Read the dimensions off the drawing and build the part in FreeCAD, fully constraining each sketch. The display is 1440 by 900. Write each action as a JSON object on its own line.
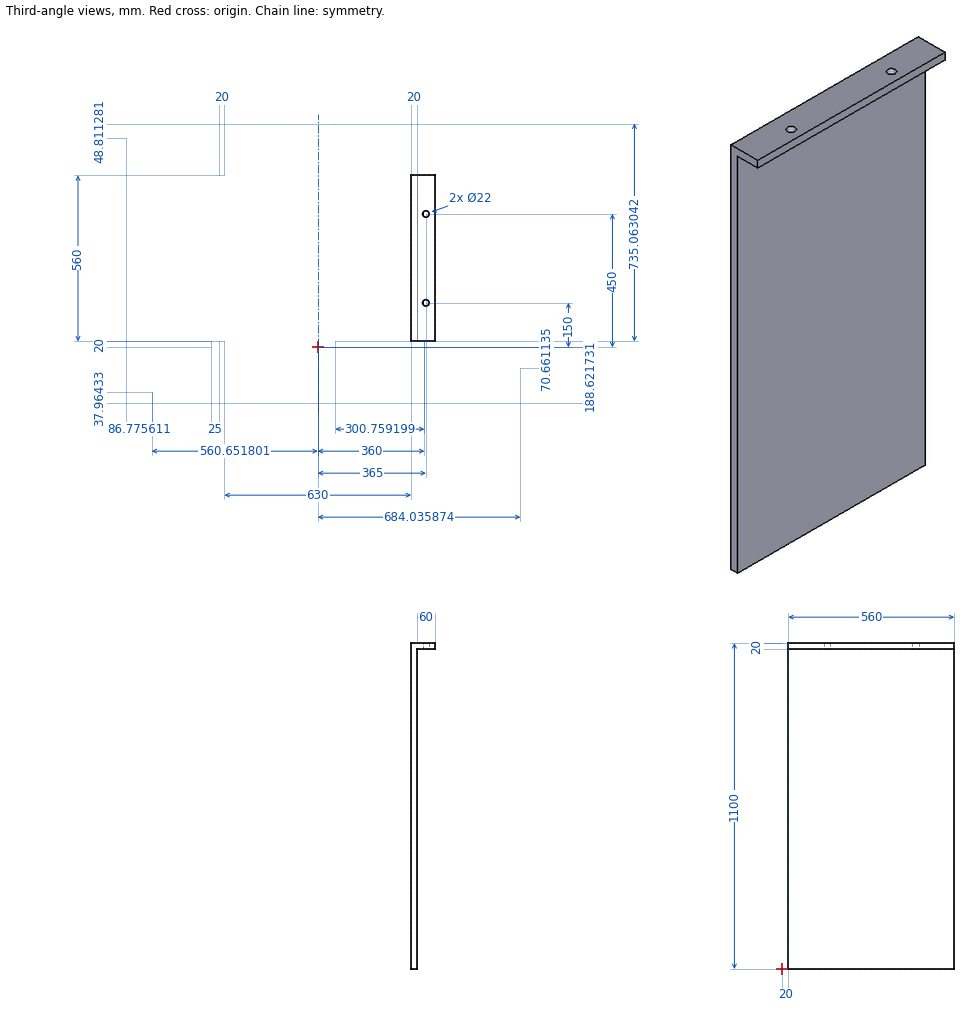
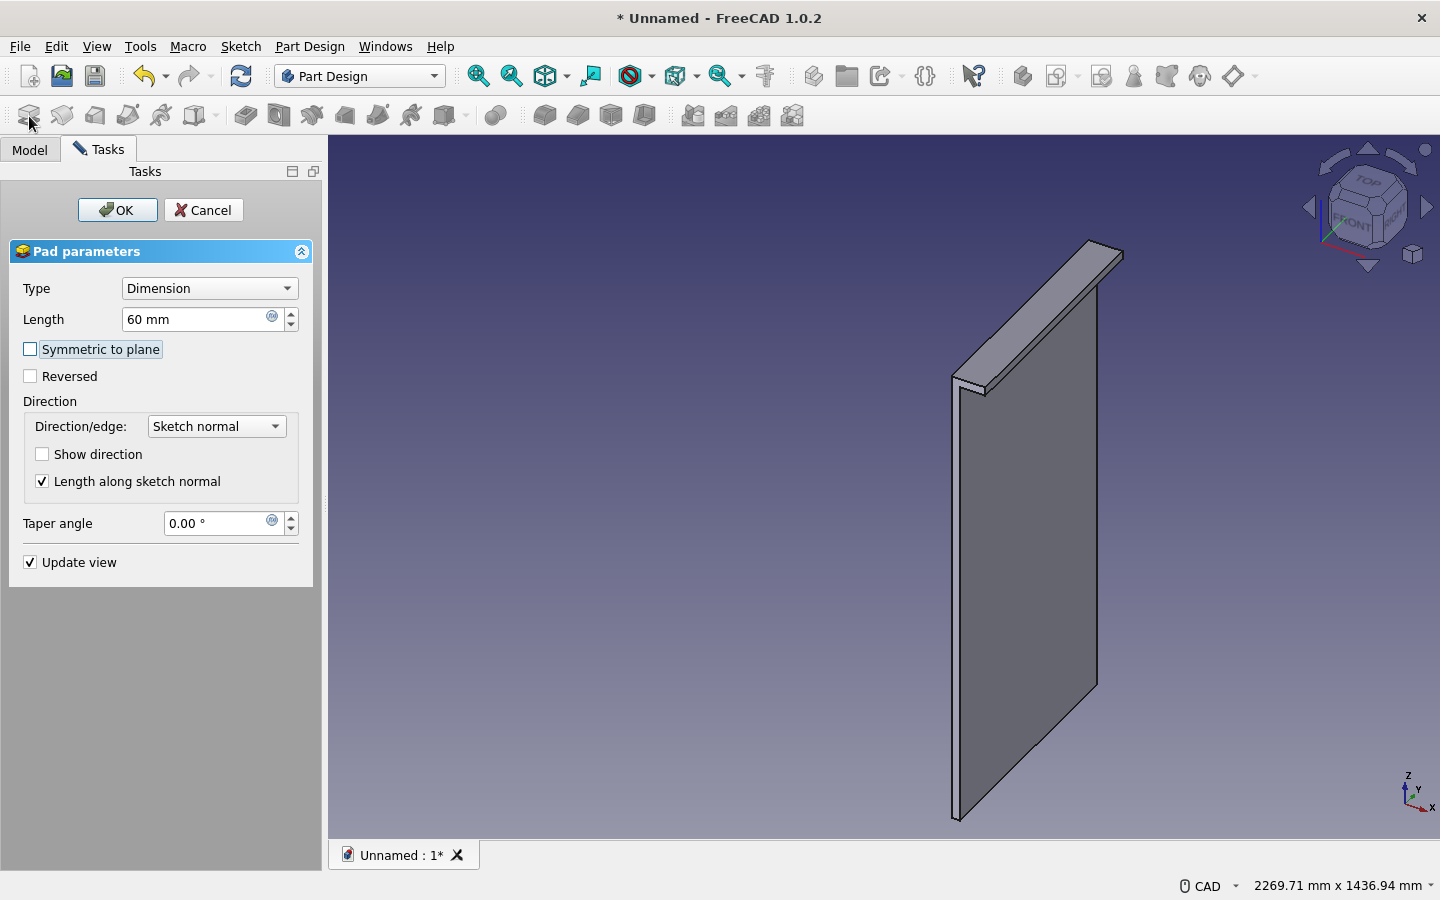
{"action": "left_click", "coordinate": [118, 210]}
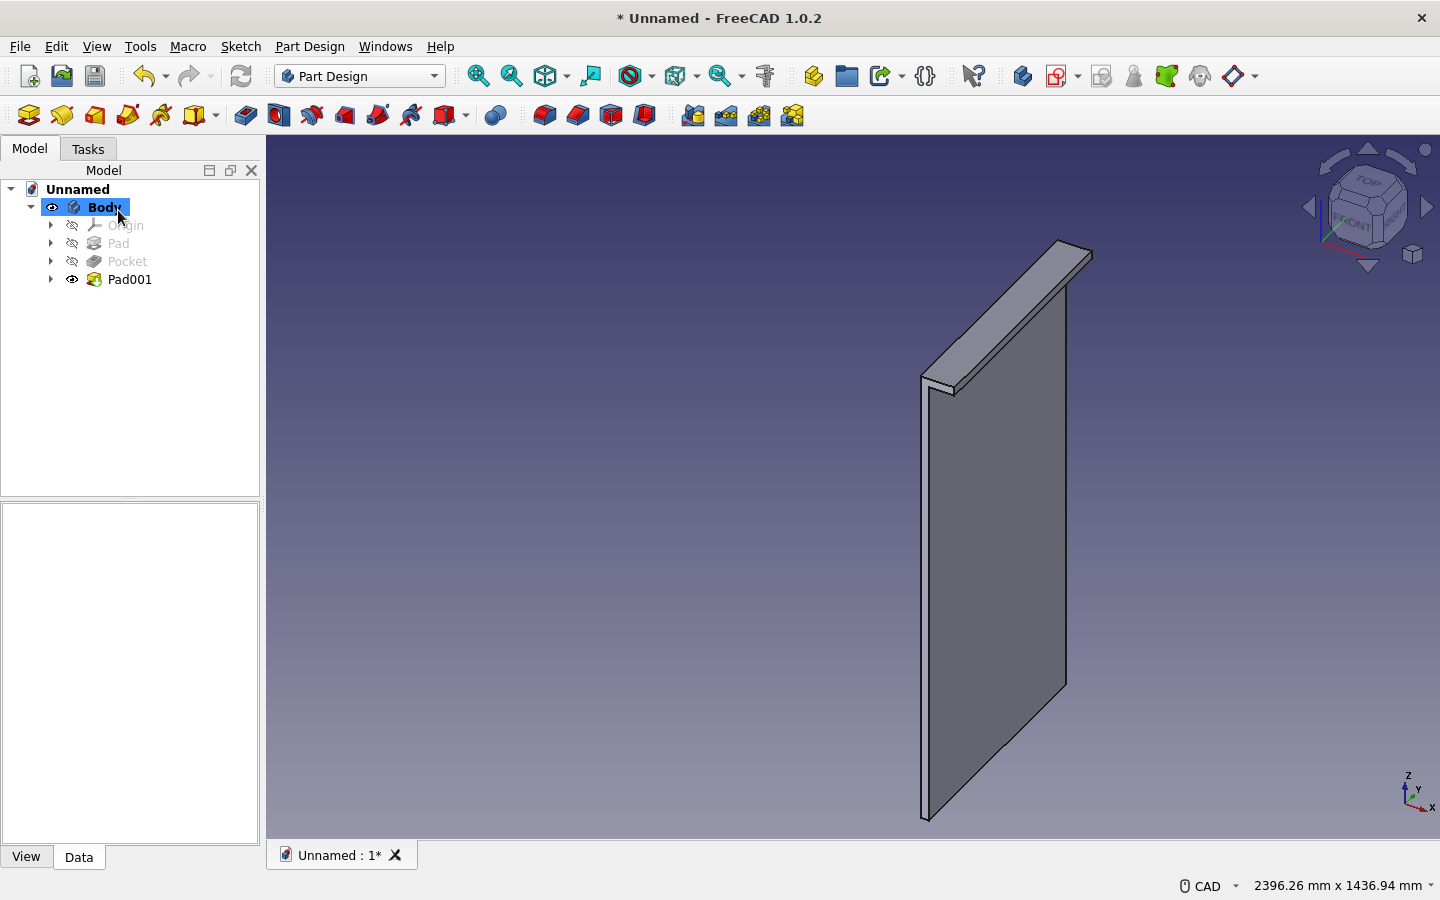
{"action": "key", "text": "5"}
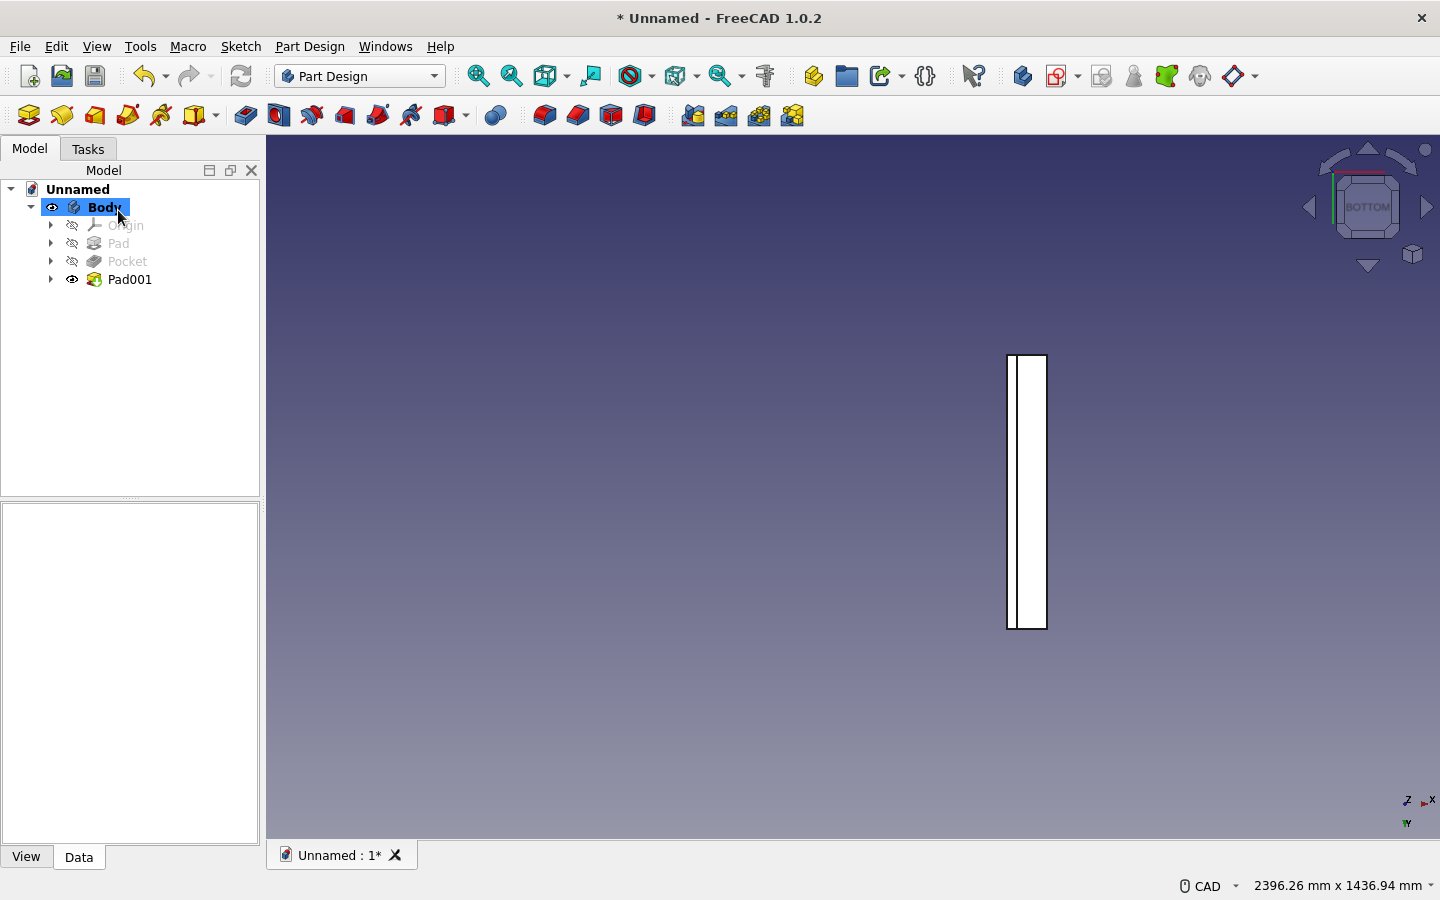
{"action": "left_click", "coordinate": [479, 76]}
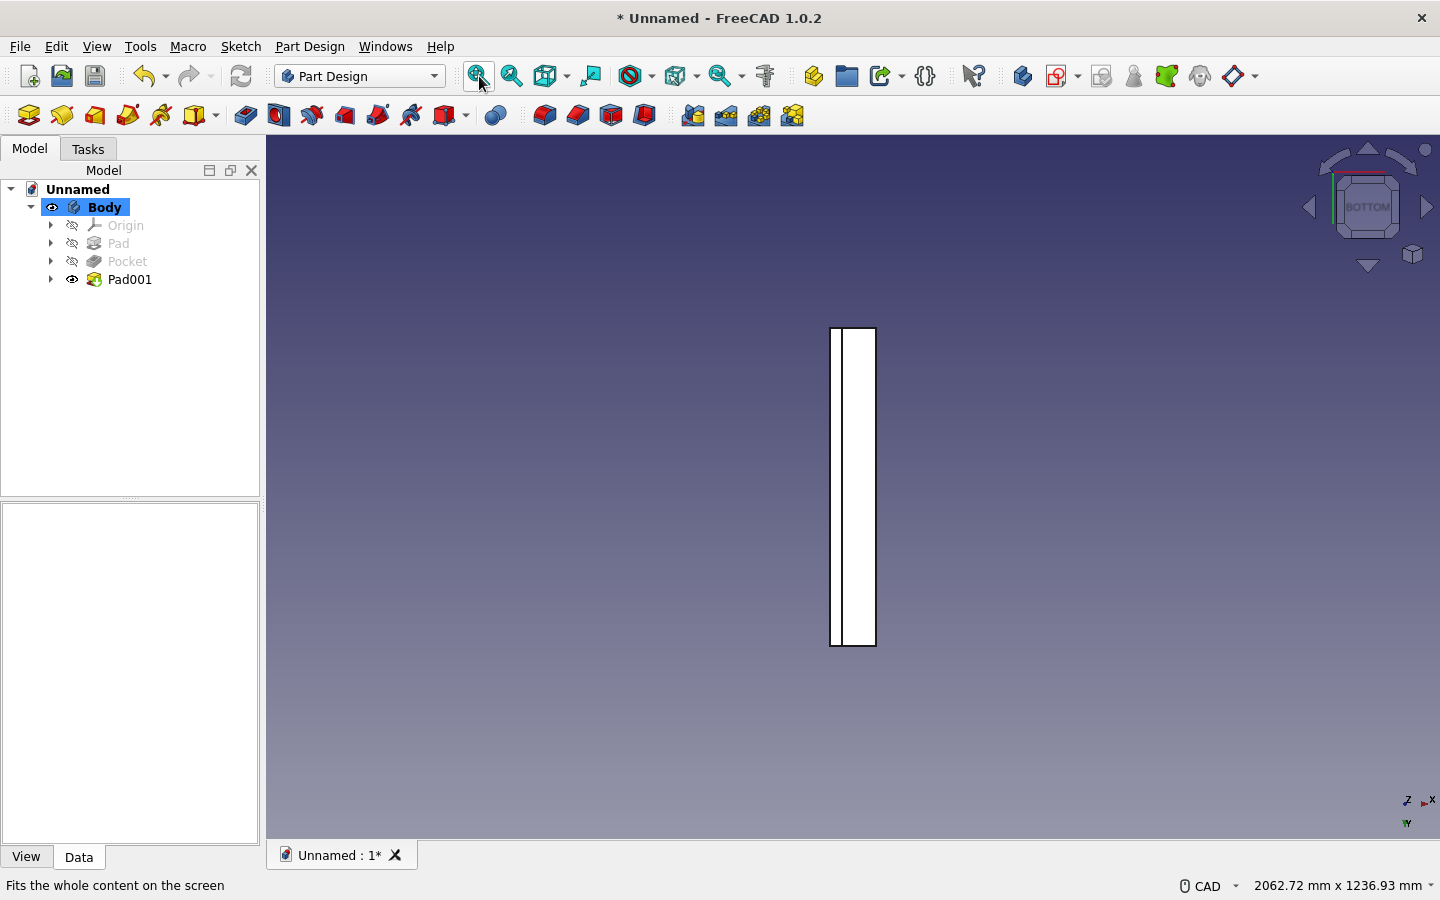
{"action": "left_click", "coordinate": [859, 623]}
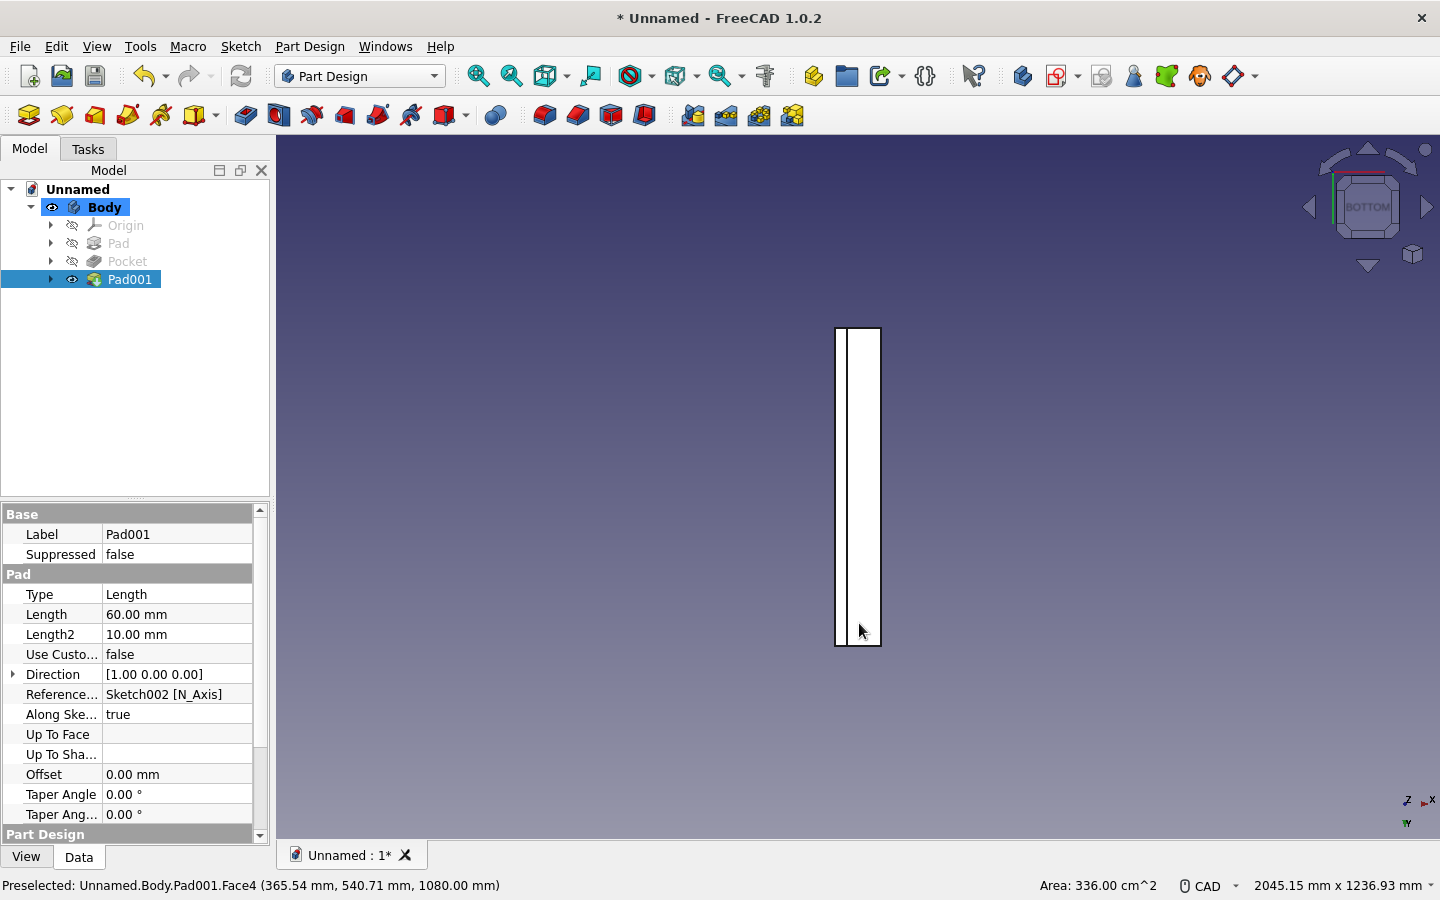
{"action": "left_click", "coordinate": [1056, 76]}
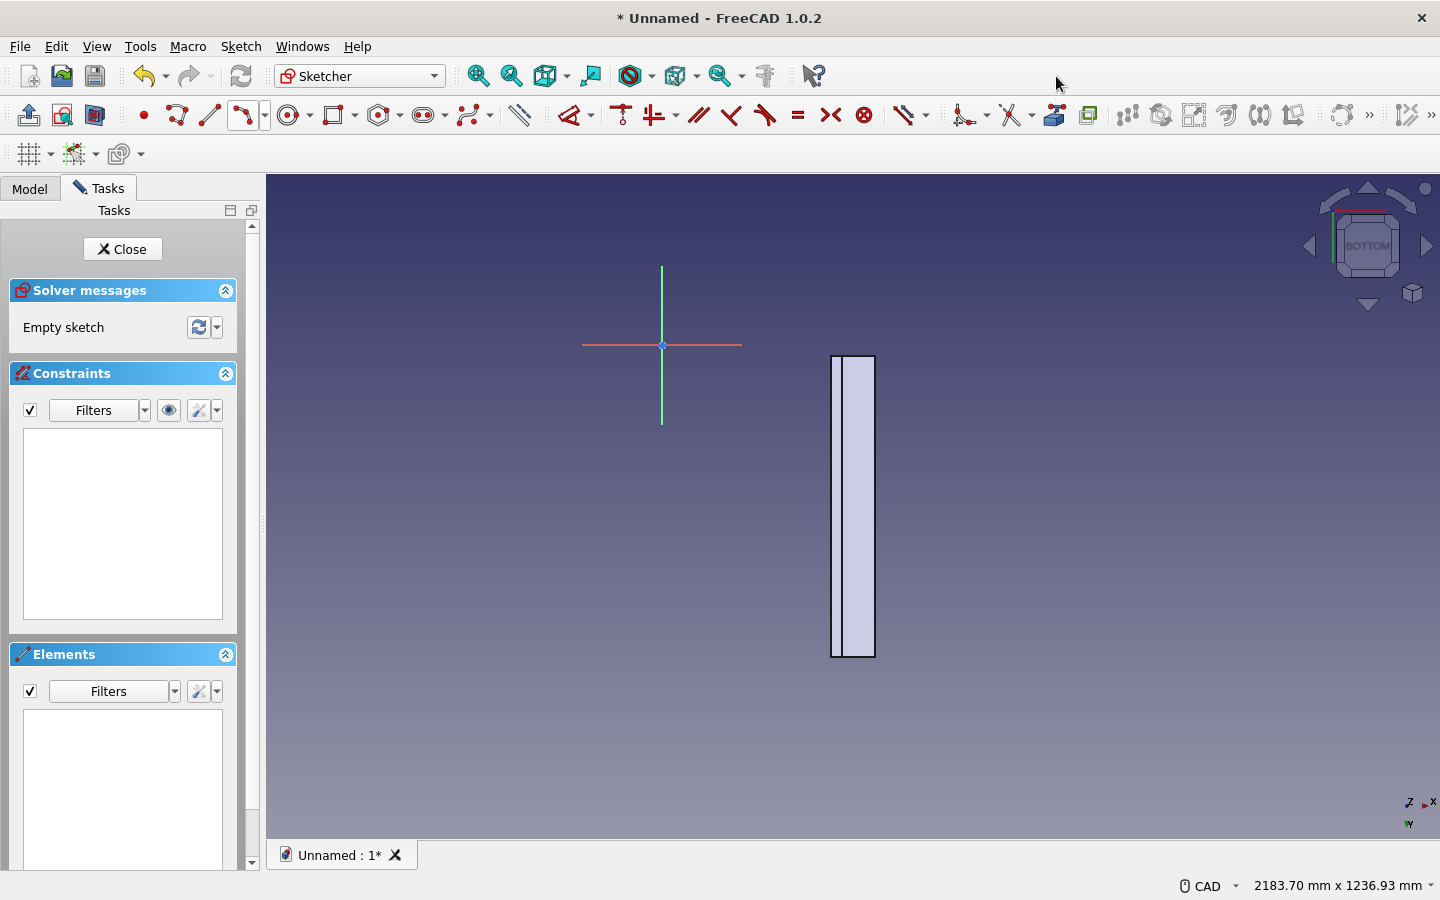
{"action": "left_click", "coordinate": [95, 116]}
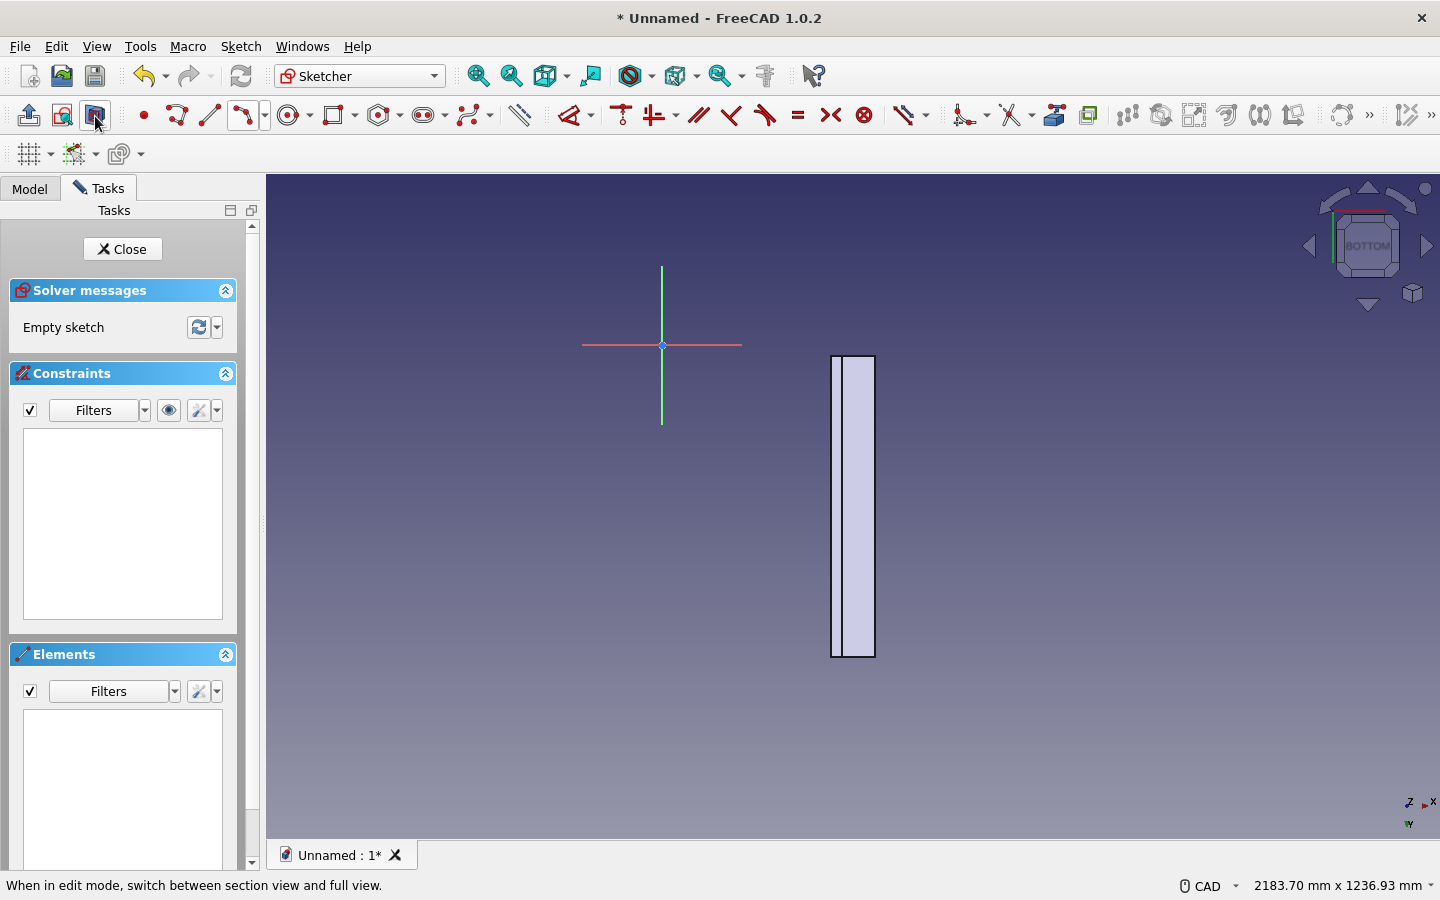
{"action": "scroll", "coordinate": [737, 424], "scroll_direction": "up", "scroll_amount": 3}